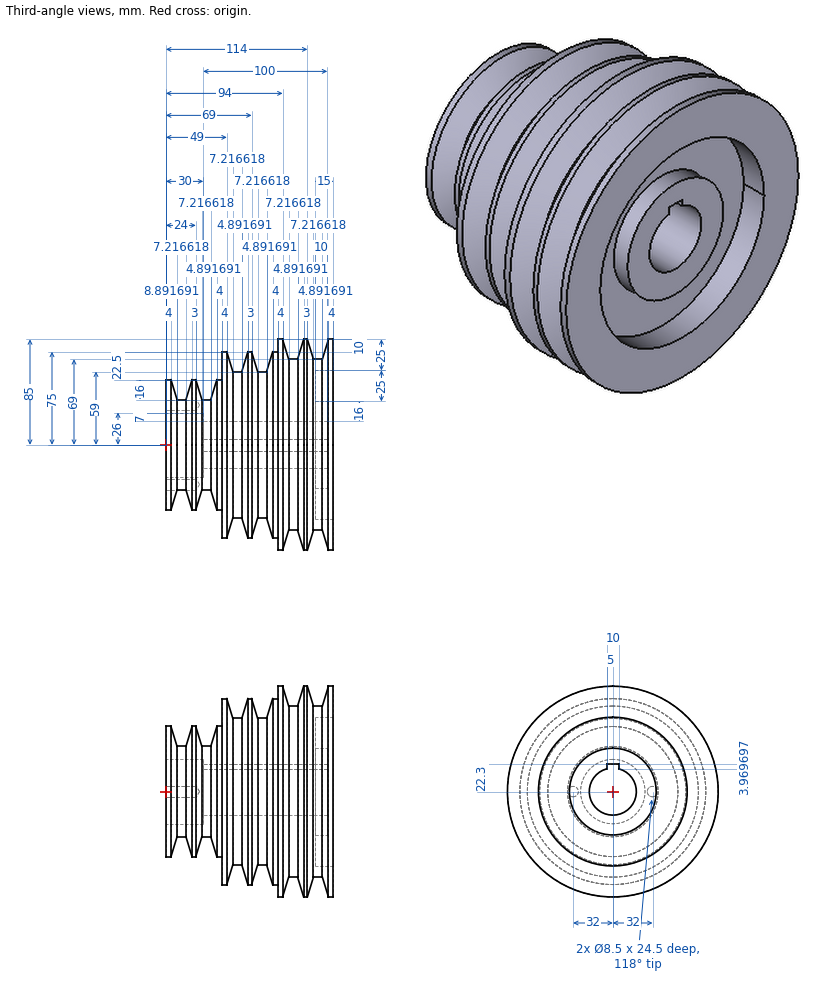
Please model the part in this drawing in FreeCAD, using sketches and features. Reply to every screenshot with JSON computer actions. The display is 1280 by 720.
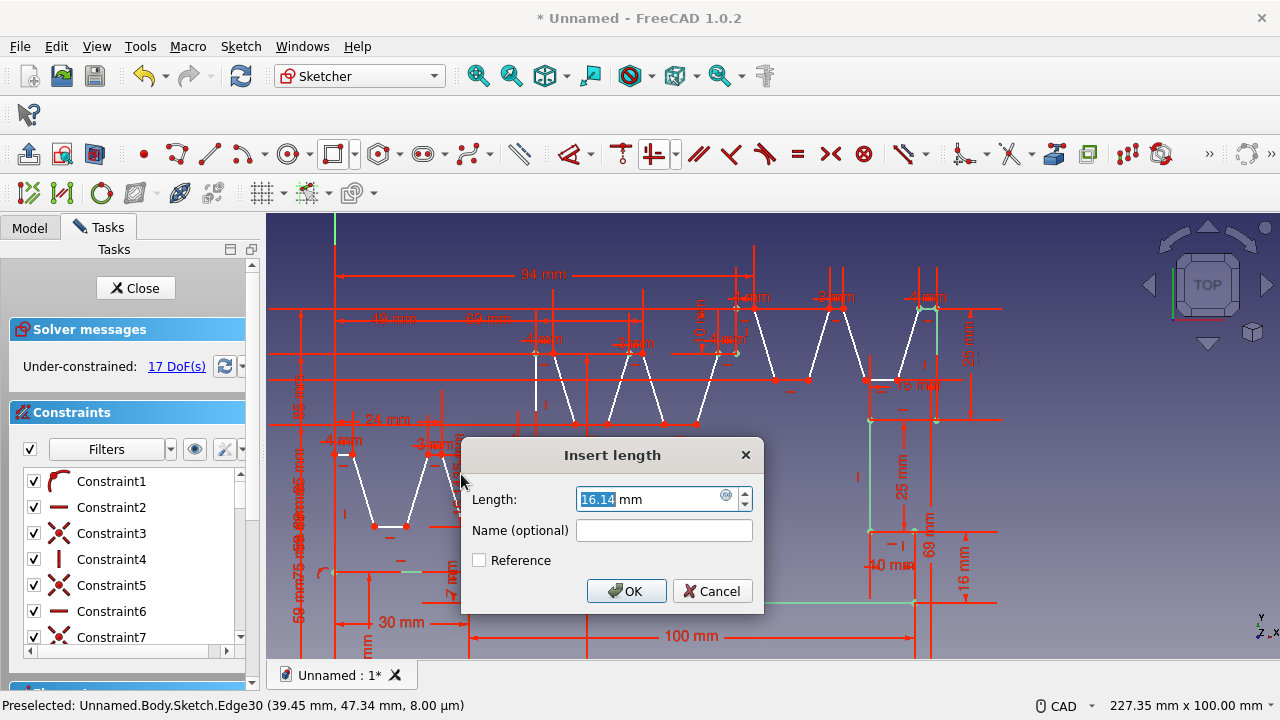
{"action": "type", "text": "16"}
{"action": "key", "text": "Return"}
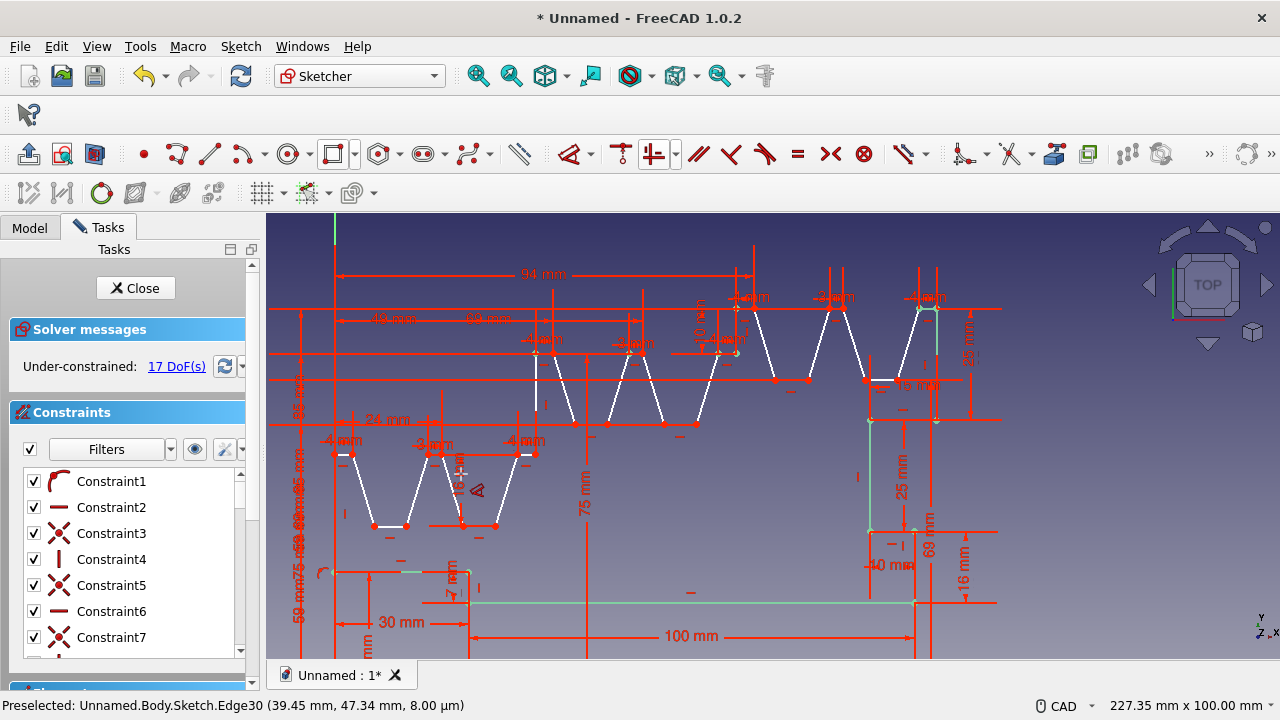
{"action": "left_click", "coordinate": [457, 505]}
{"action": "left_click", "coordinate": [384, 490]}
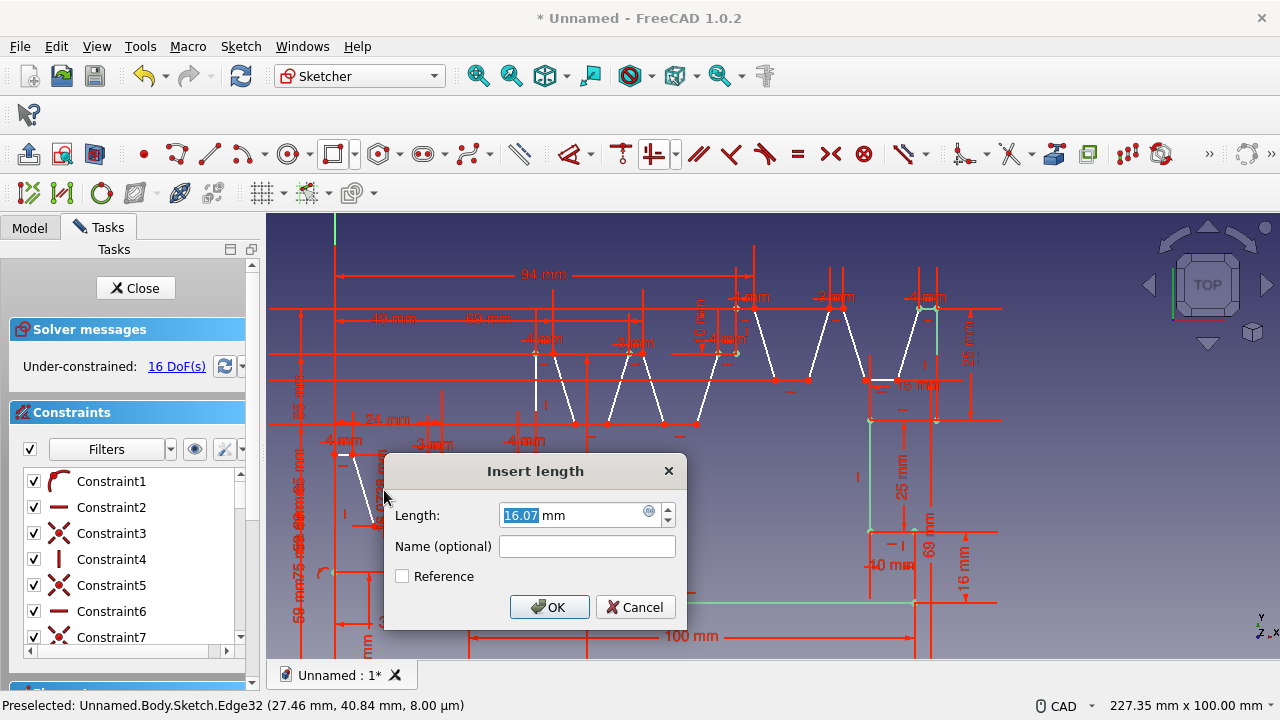
{"action": "type", "text": "16"}
{"action": "key", "text": "Return"}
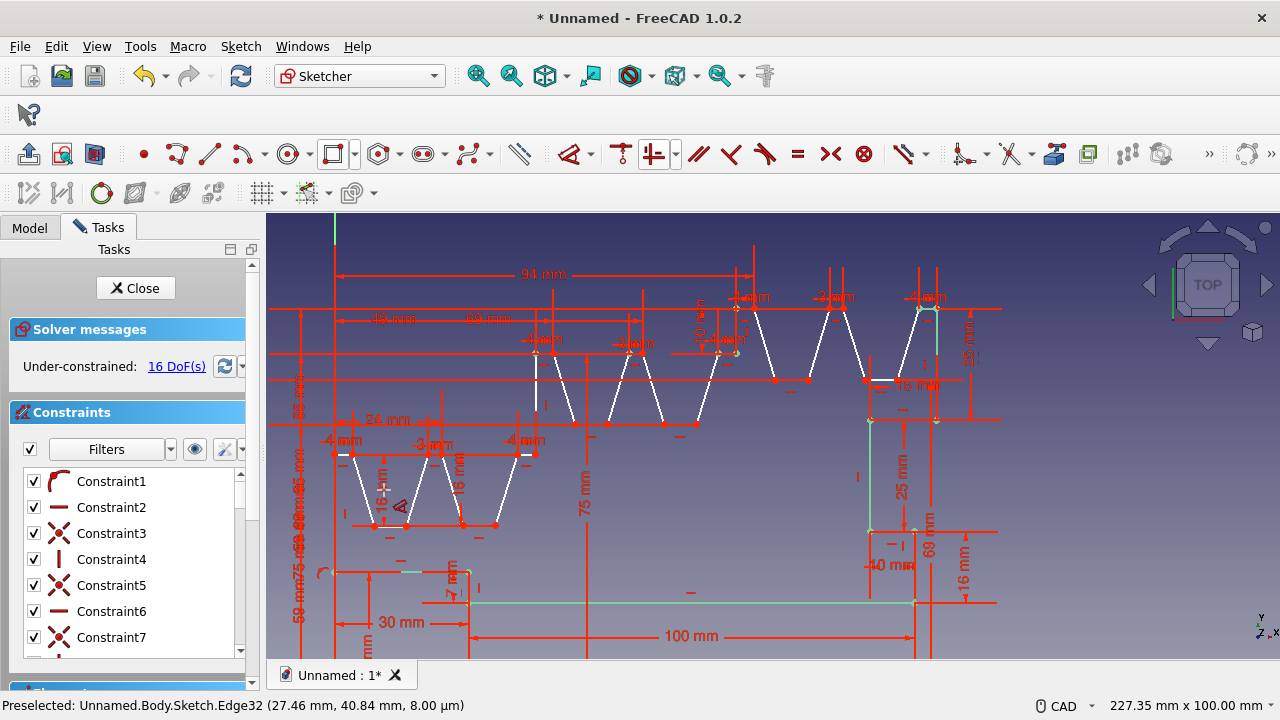
{"action": "left_click", "coordinate": [422, 476]}
{"action": "left_click", "coordinate": [486, 507]}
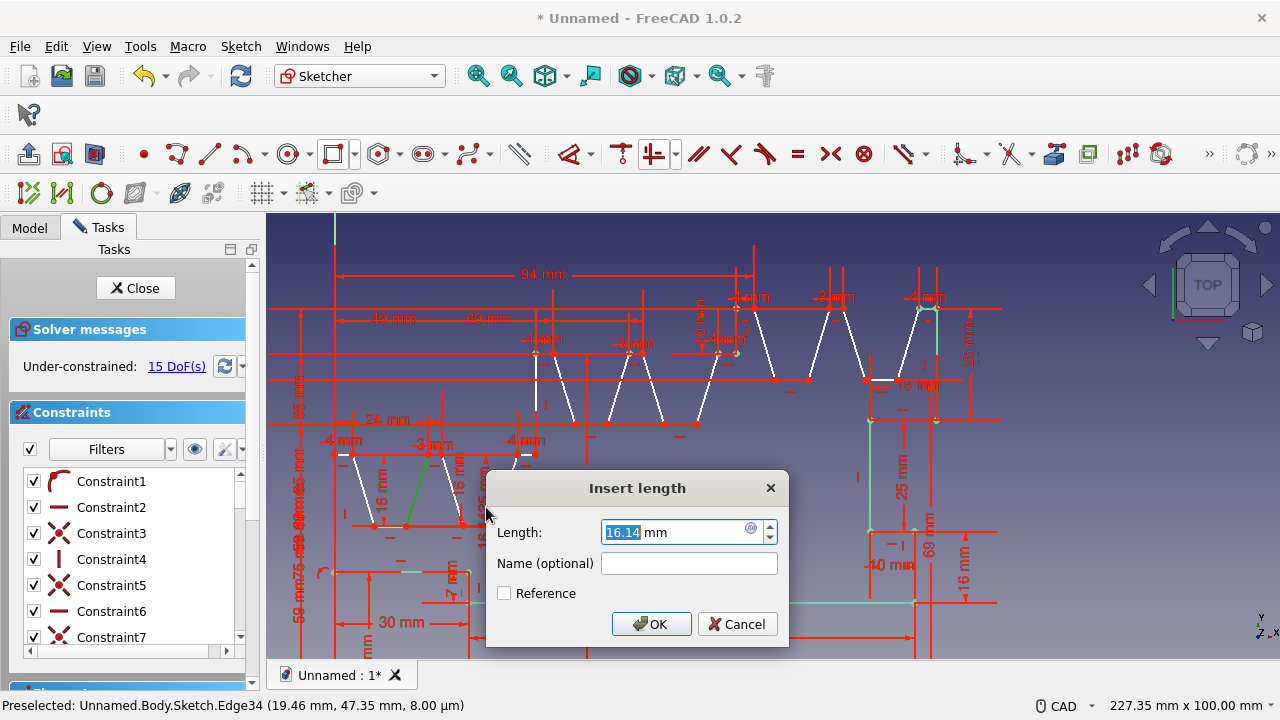
{"action": "type", "text": "16"}
{"action": "key", "text": "Return"}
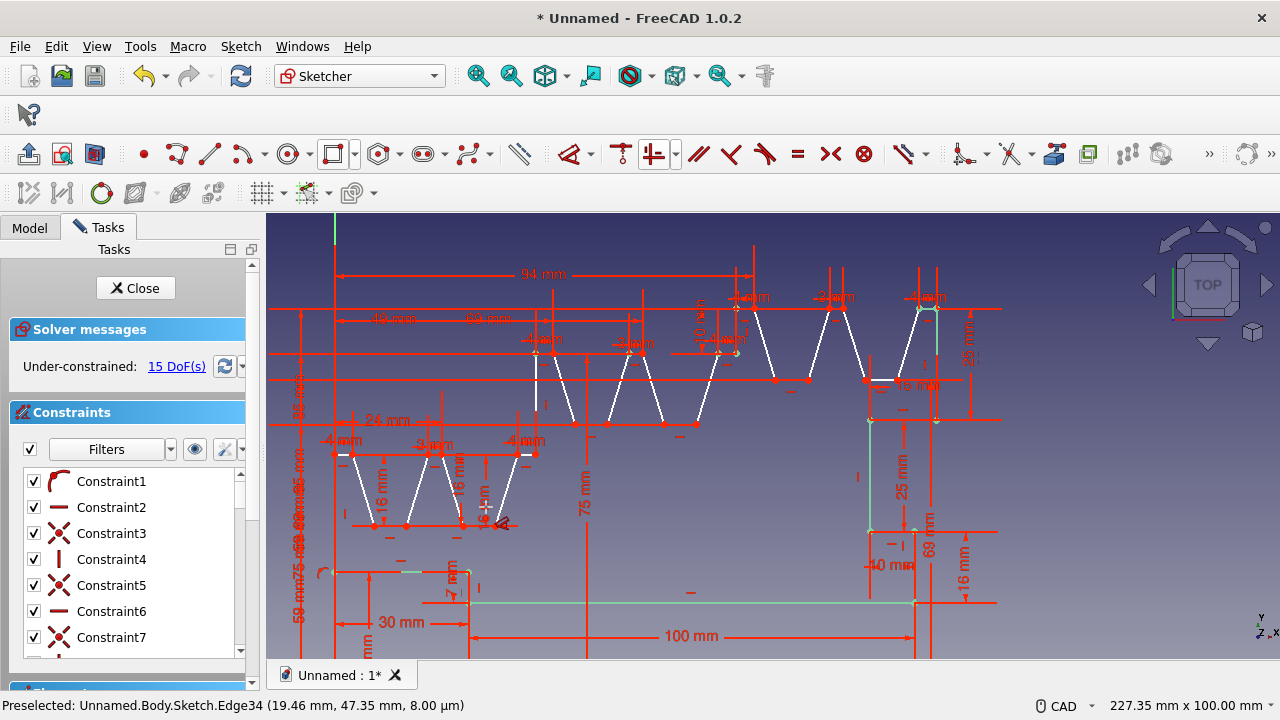
{"action": "left_click", "coordinate": [368, 505]}
{"action": "left_click", "coordinate": [554, 465]}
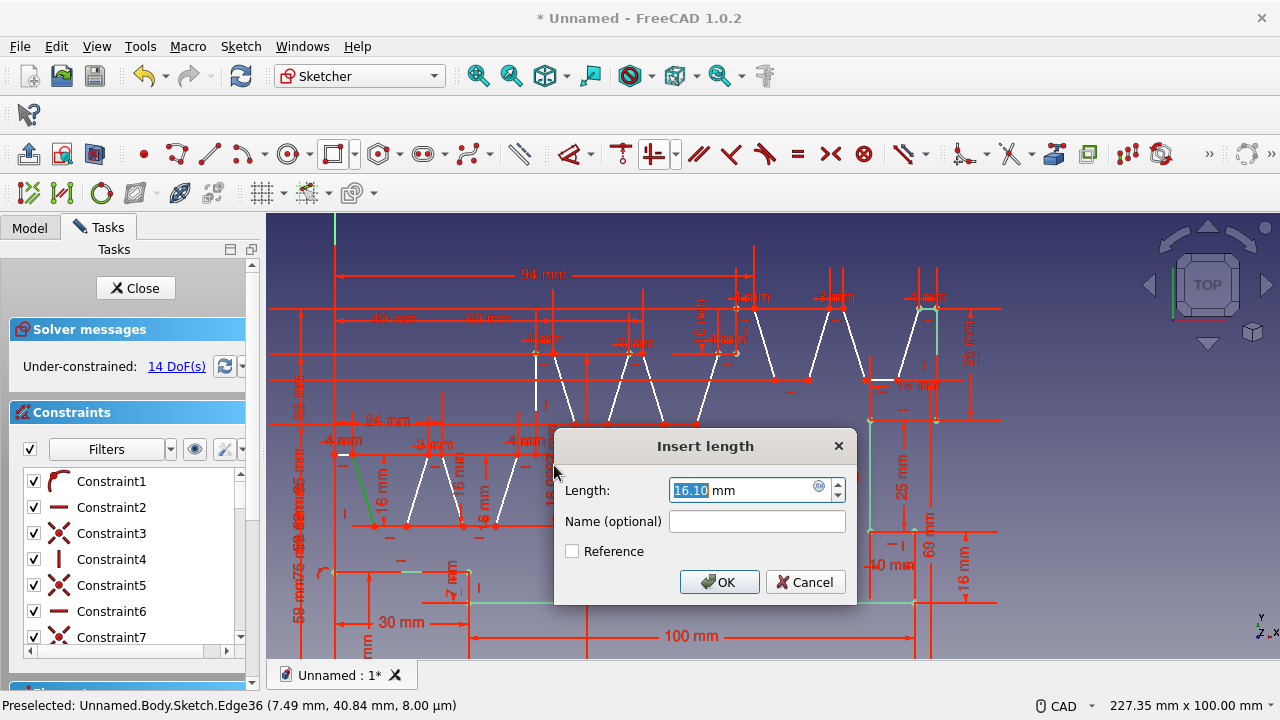
{"action": "type", "text": "16"}
{"action": "key", "text": "Return"}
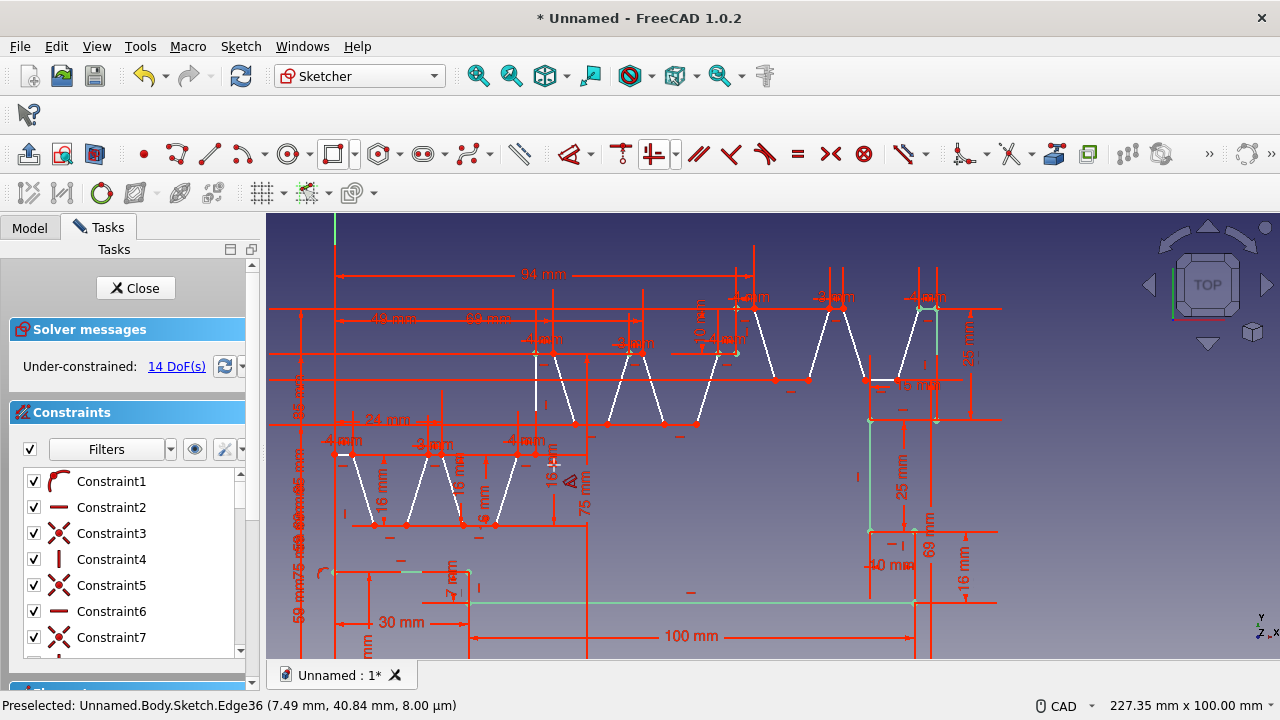
{"action": "left_click", "coordinate": [536, 384]}
{"action": "left_click", "coordinate": [502, 404]}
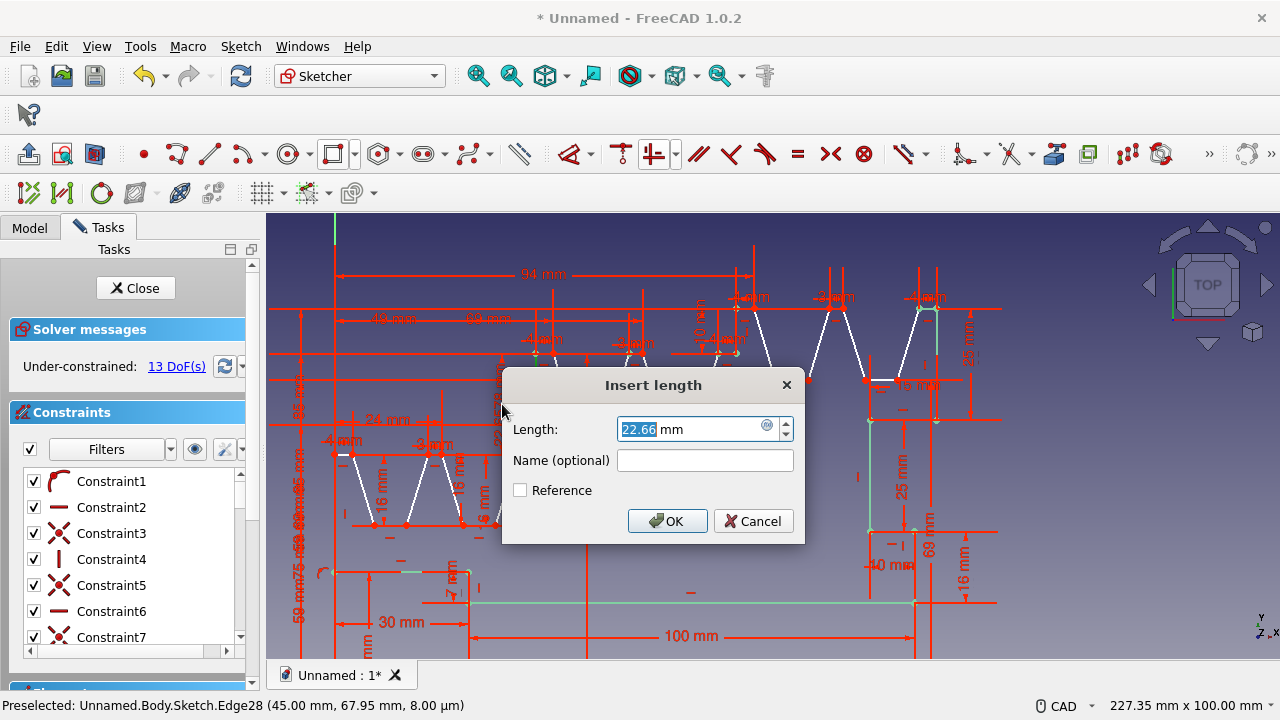
{"action": "type", "text": "22.5"}
{"action": "key", "text": "Return"}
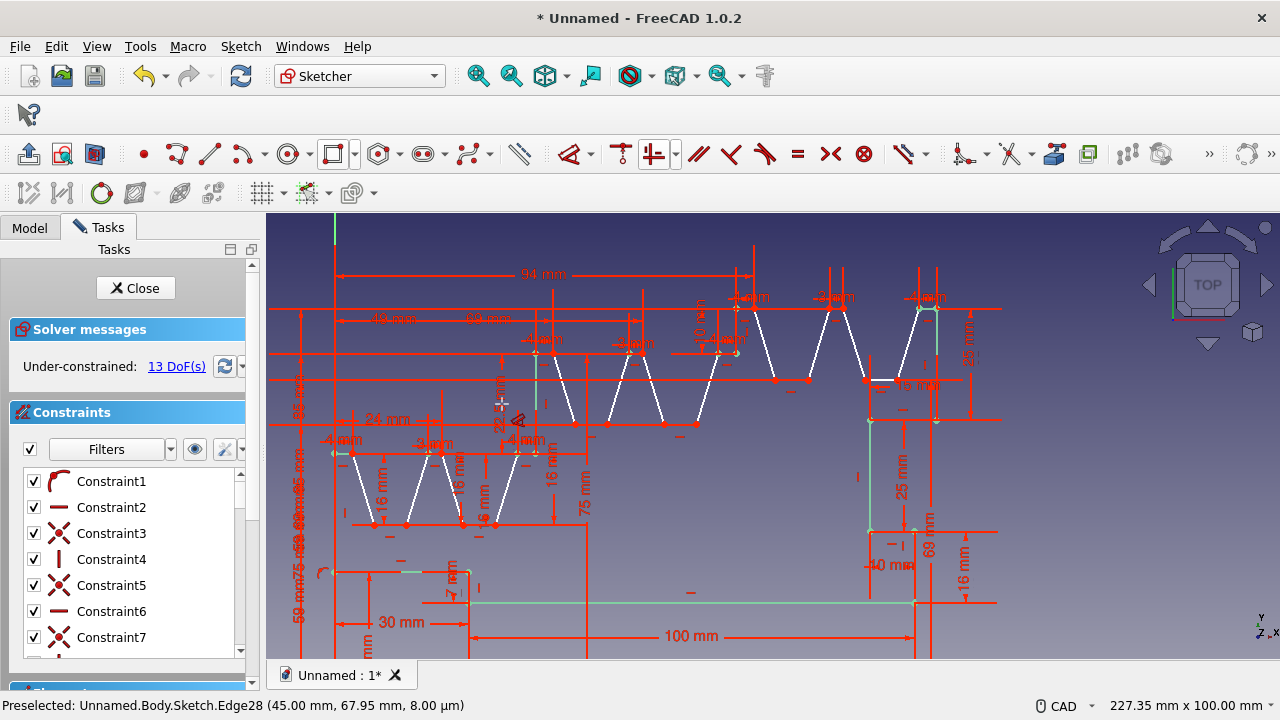
{"action": "left_click", "coordinate": [843, 309]}
{"action": "left_click", "coordinate": [472, 275]}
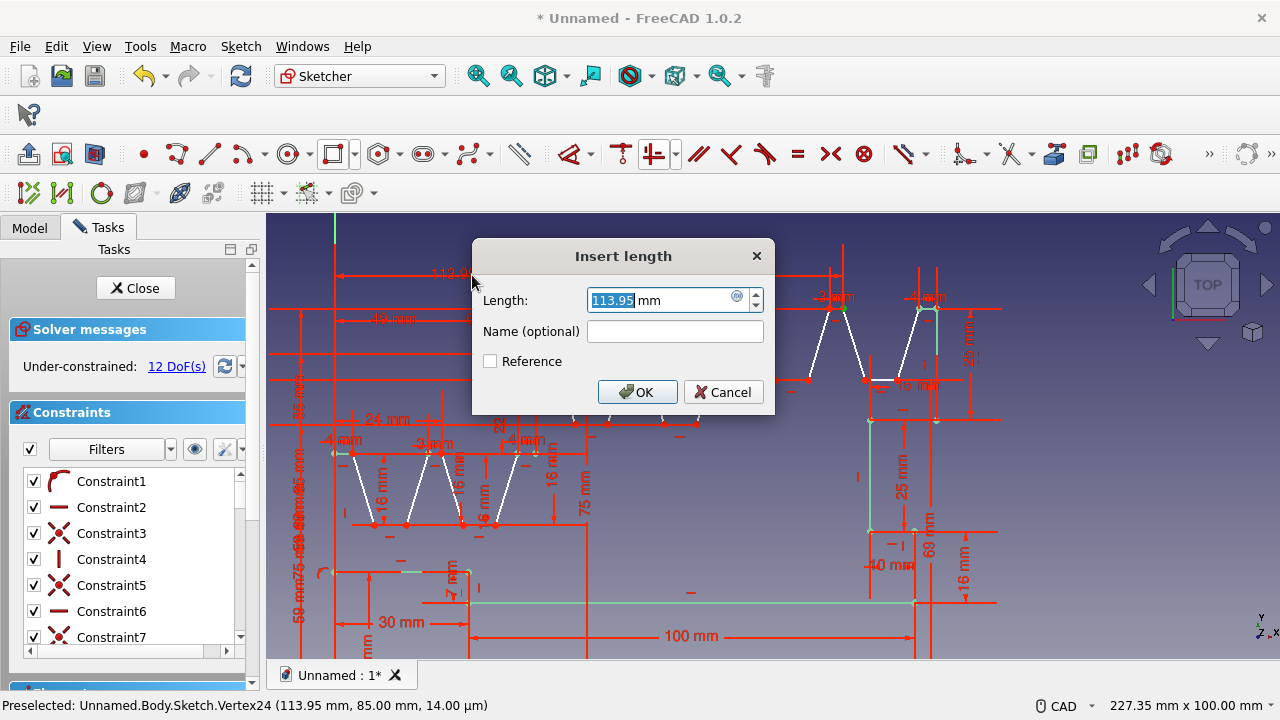
{"action": "type", "text": "114"}
{"action": "key", "text": "Return"}